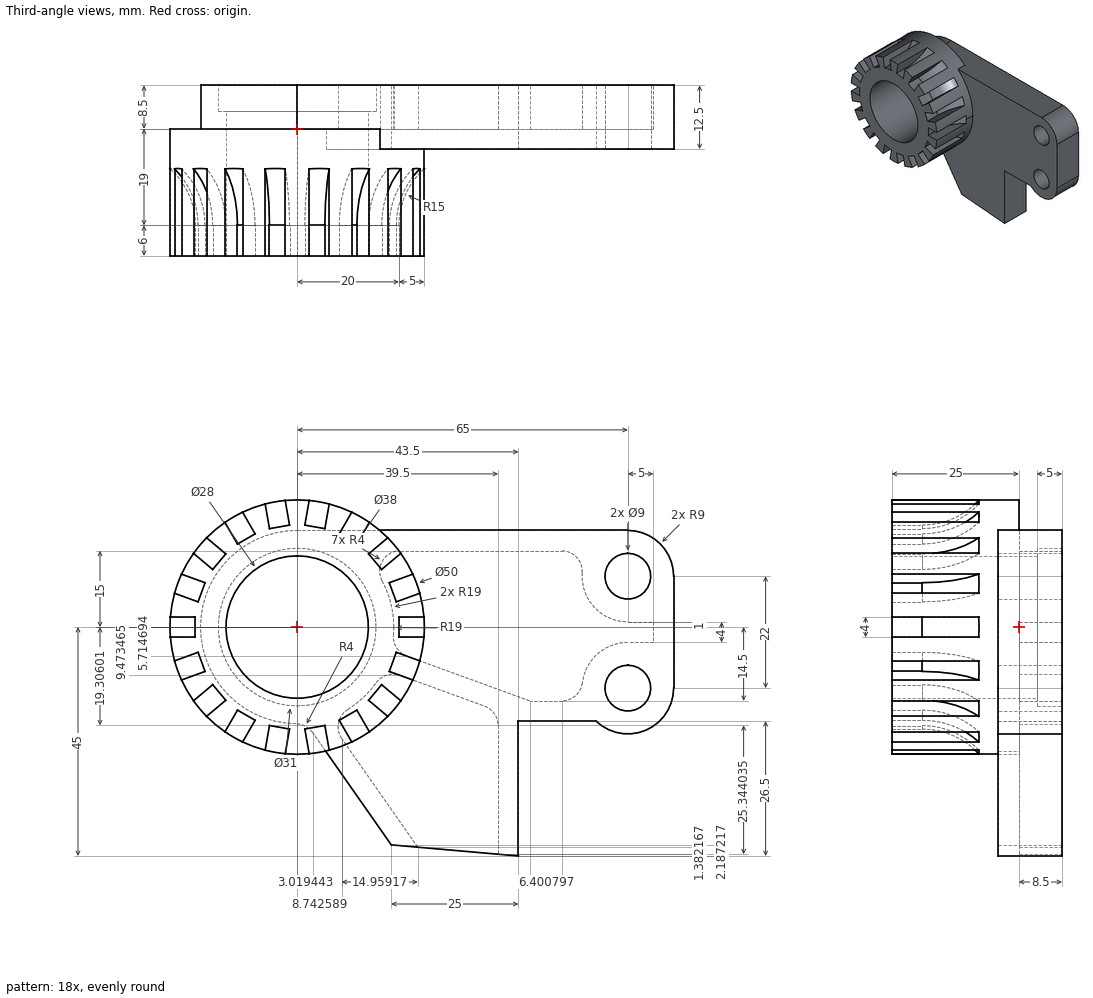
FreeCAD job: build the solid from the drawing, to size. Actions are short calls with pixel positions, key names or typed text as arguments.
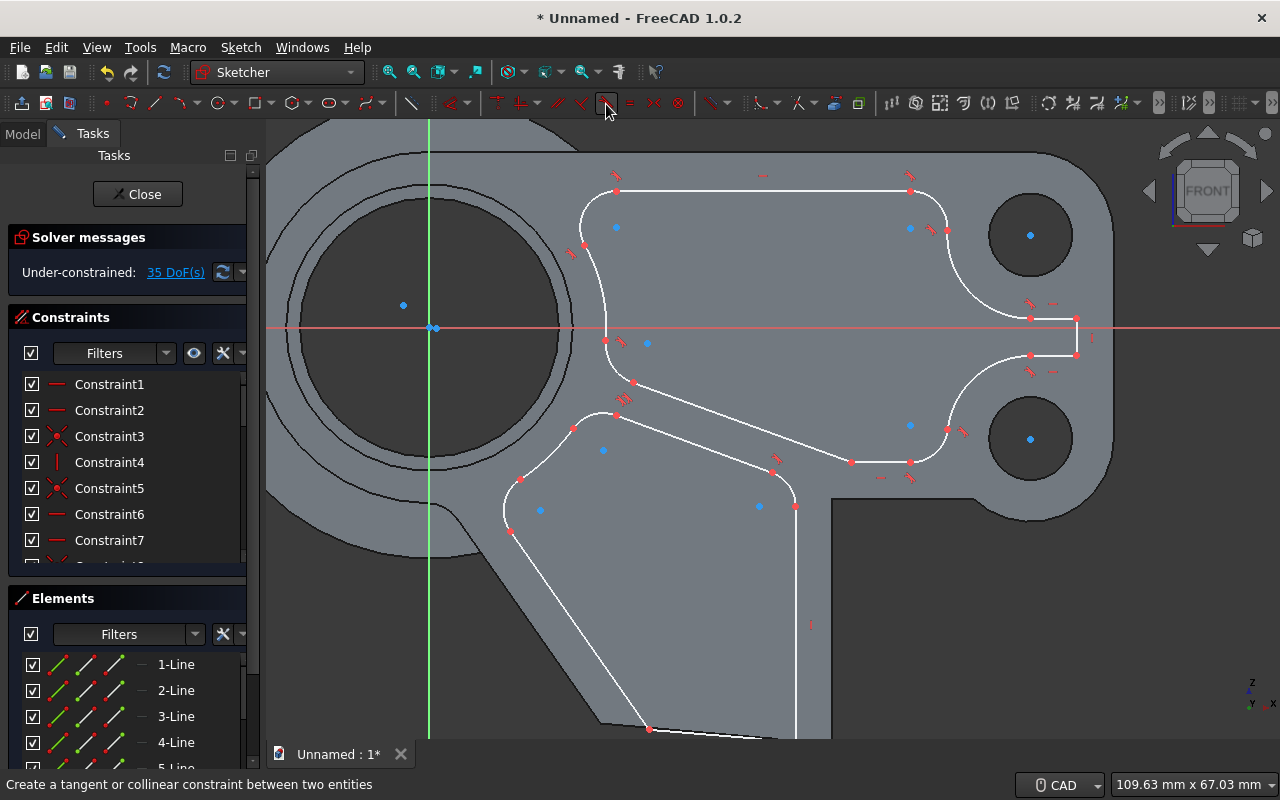
click(796, 577)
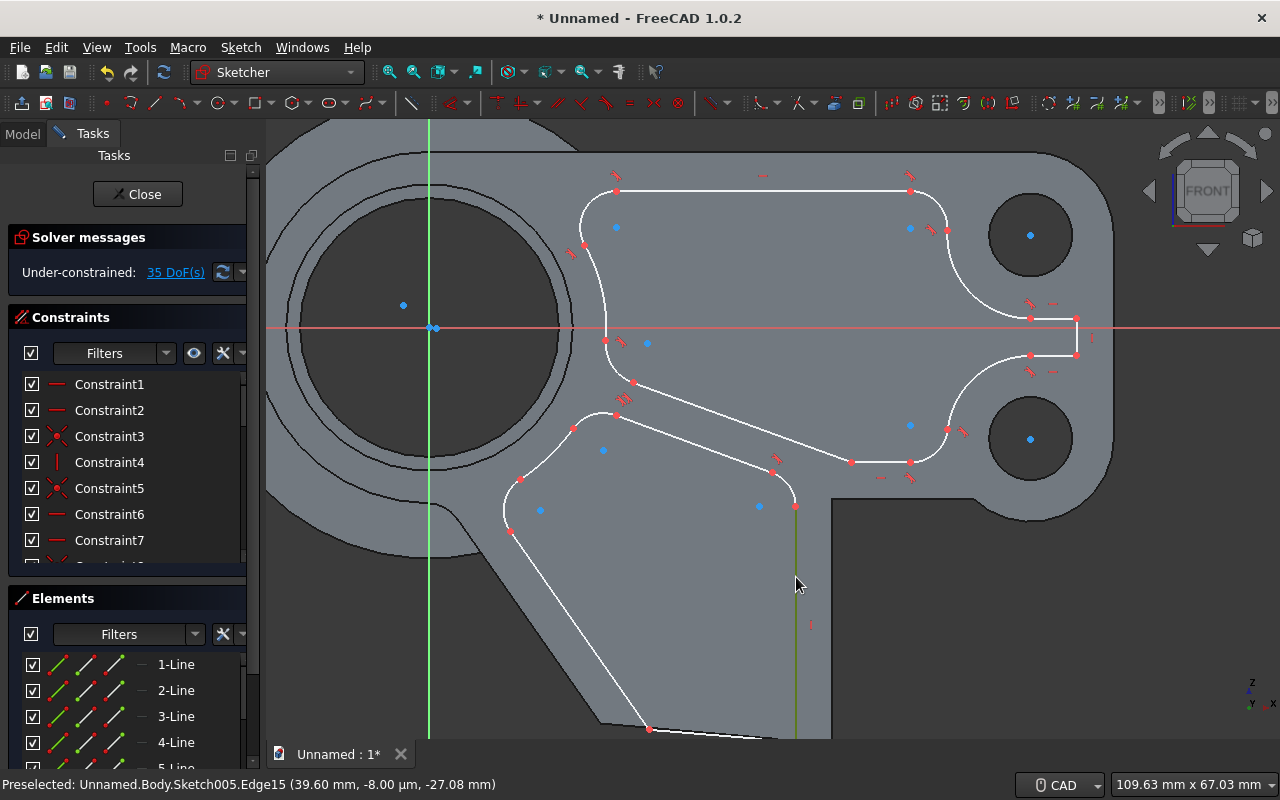
click(793, 494)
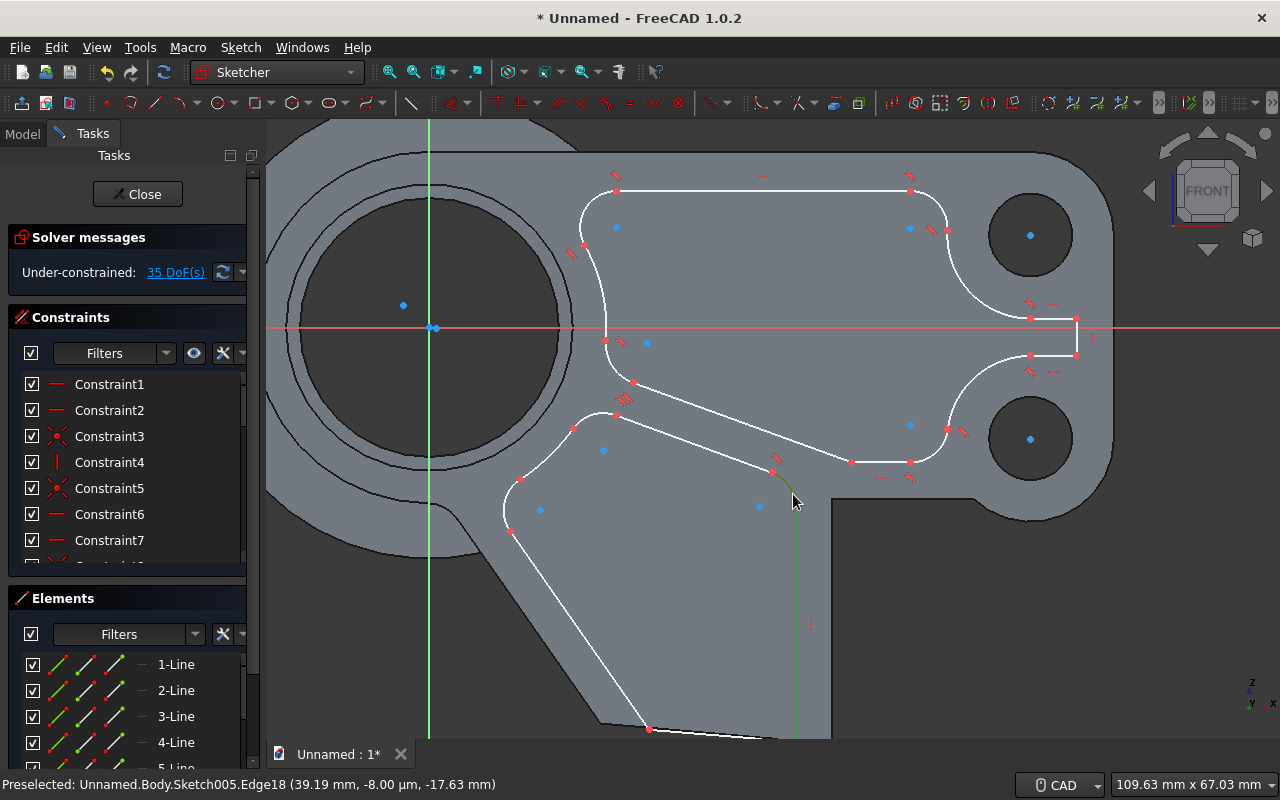
click(606, 104)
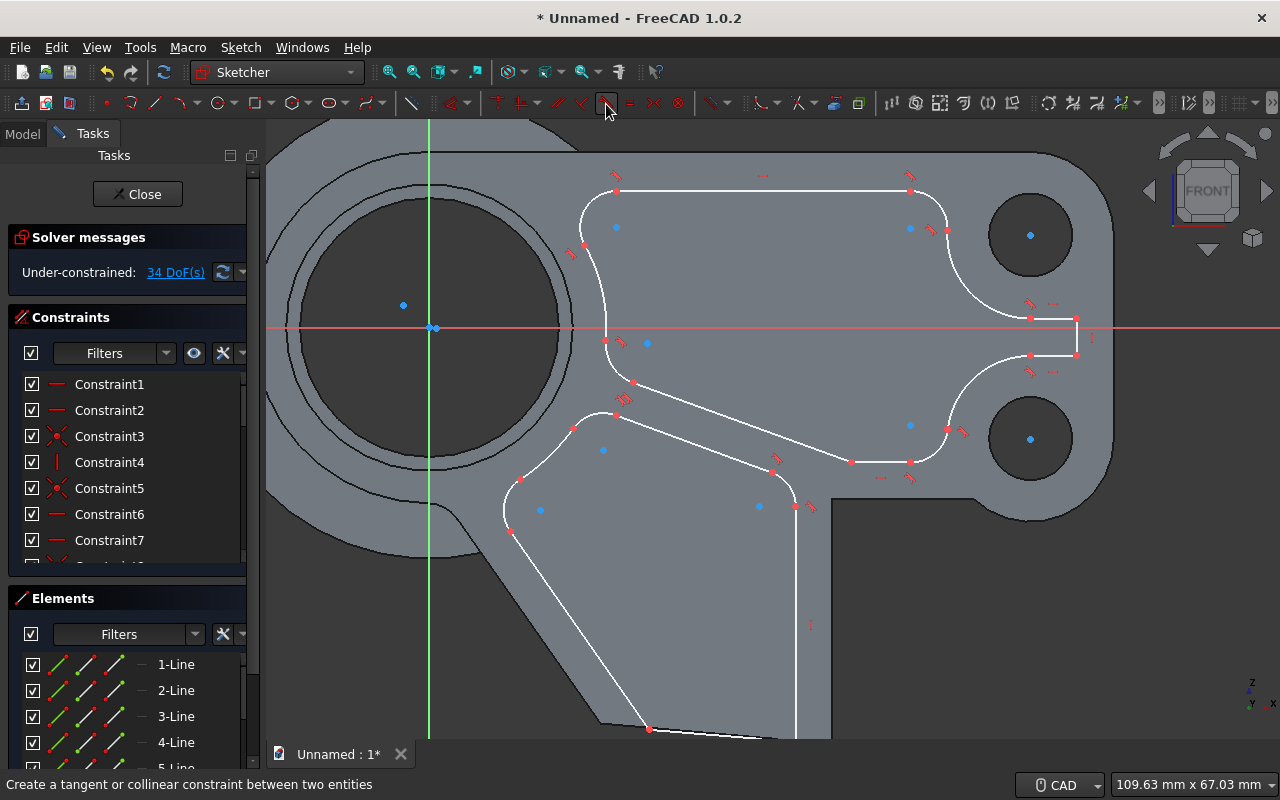
click(608, 670)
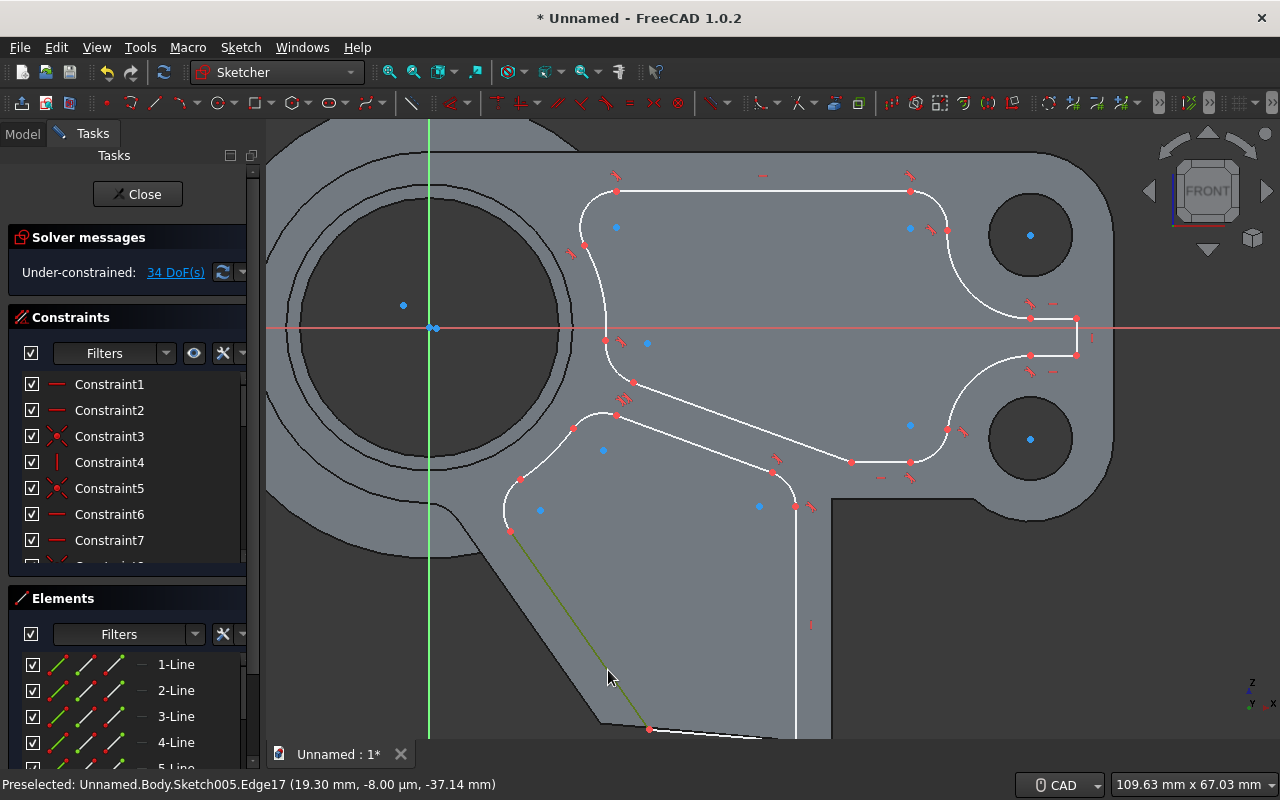
click(509, 492)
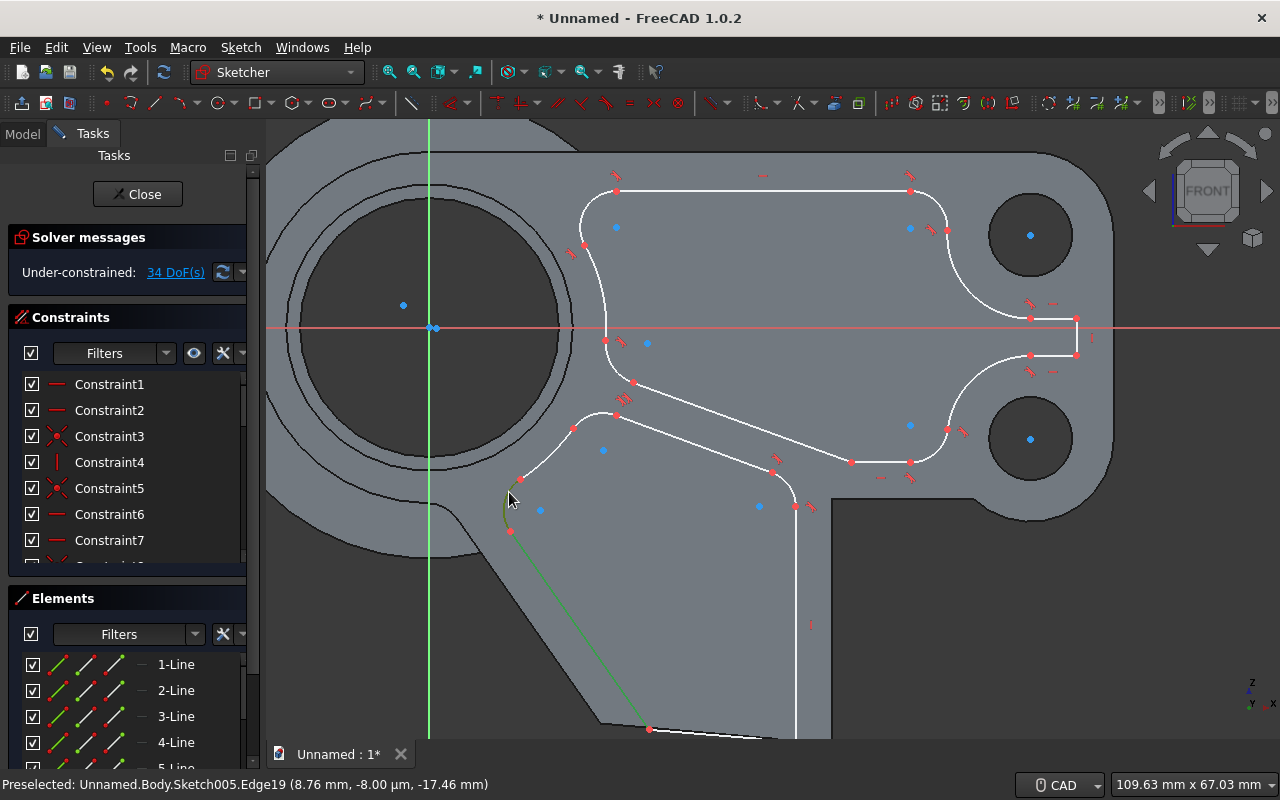
click(606, 104)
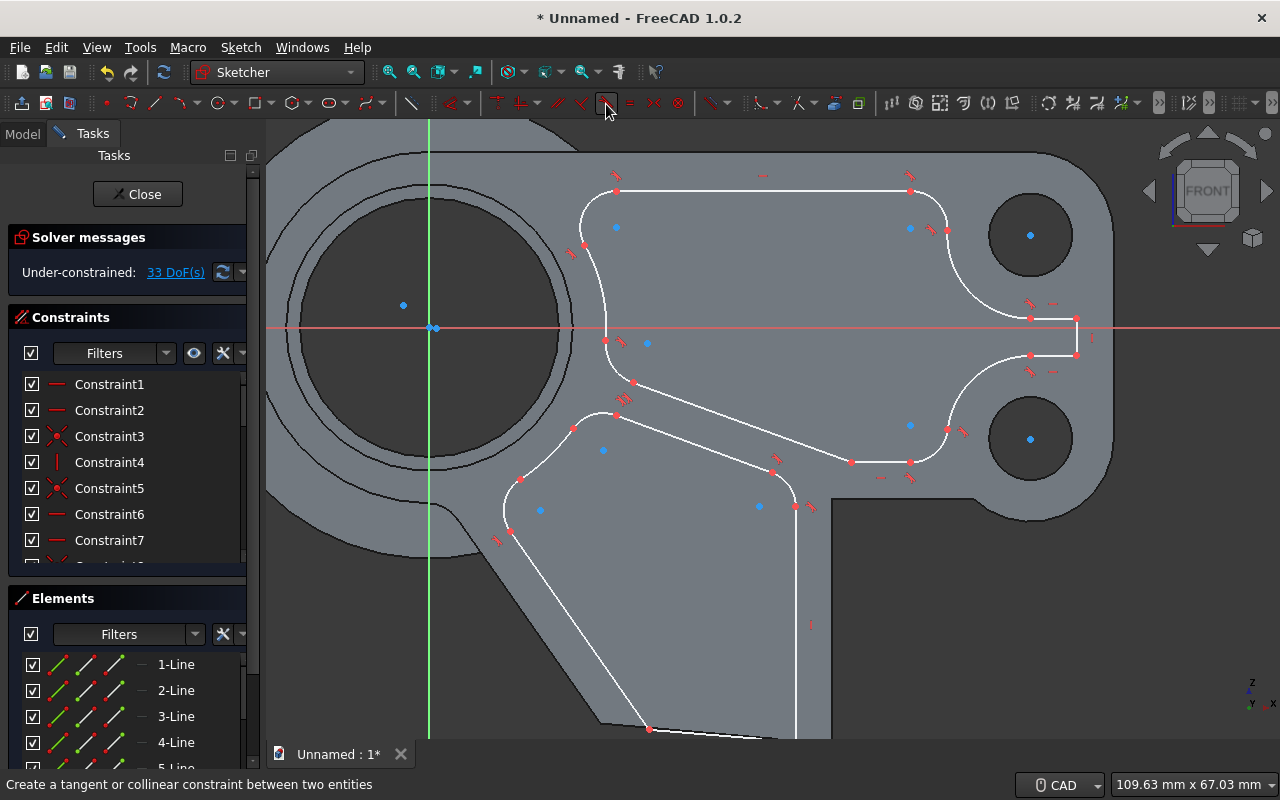
click(509, 492)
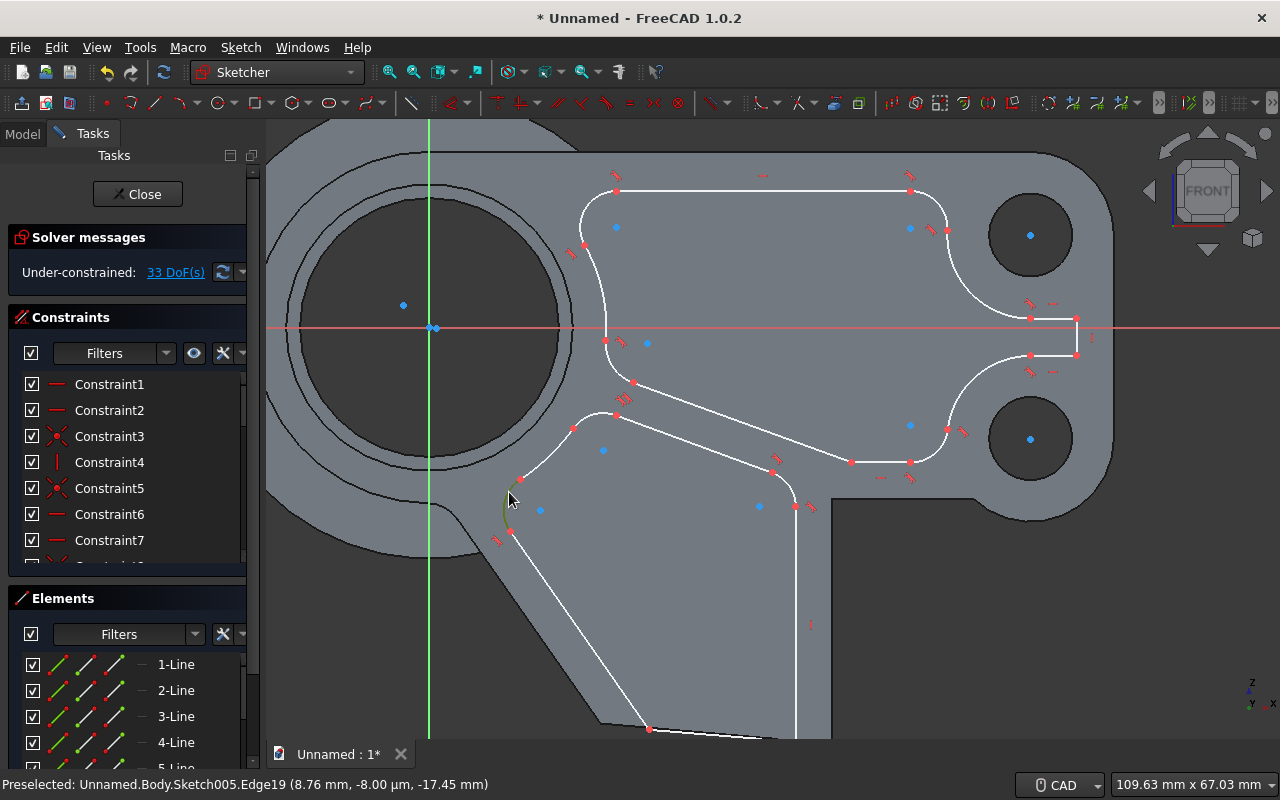
click(538, 466)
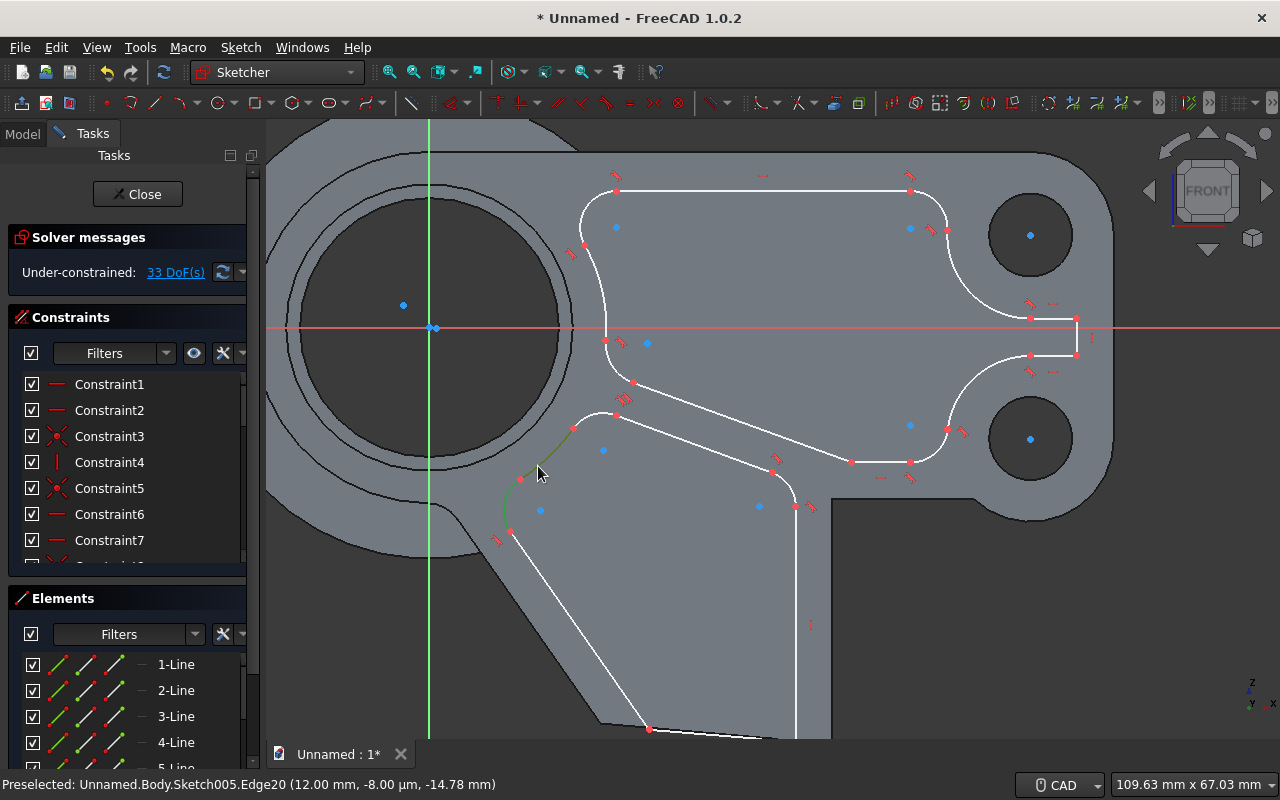
click(606, 104)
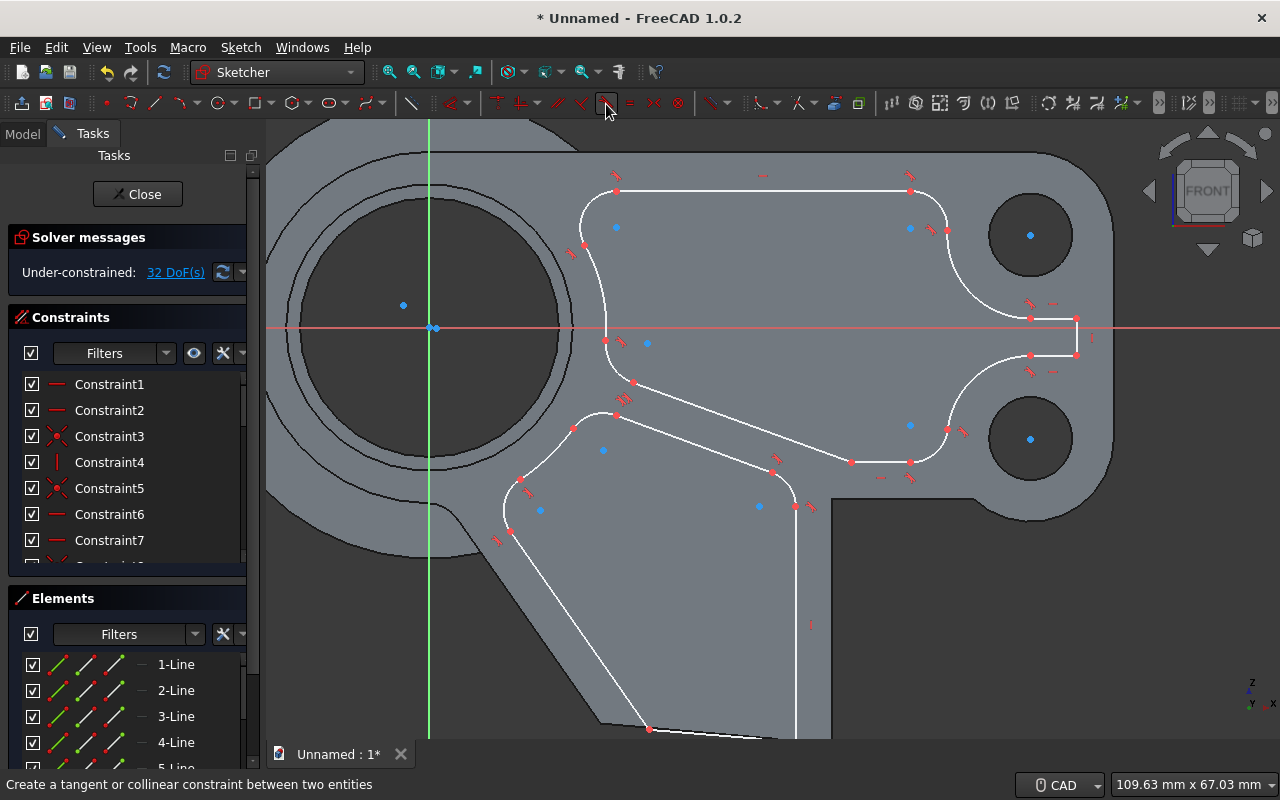
click(538, 467)